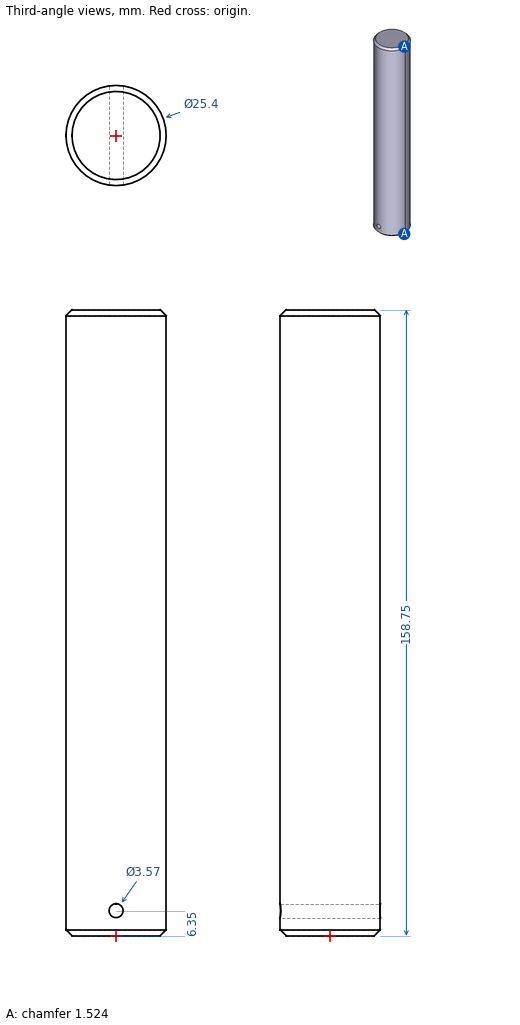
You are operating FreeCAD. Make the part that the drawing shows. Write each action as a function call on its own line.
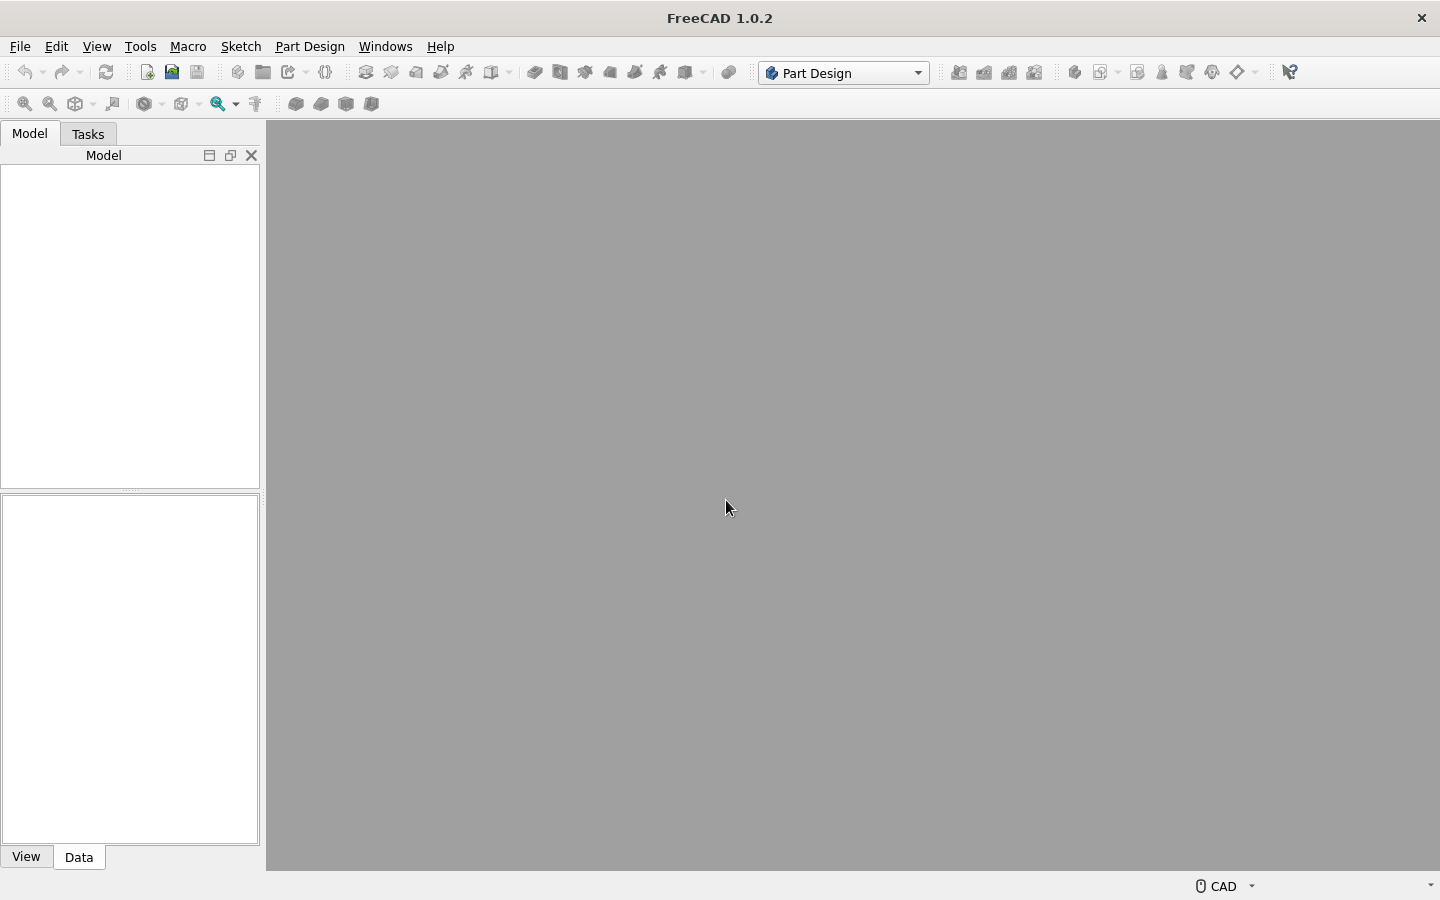
key(ctrl+n)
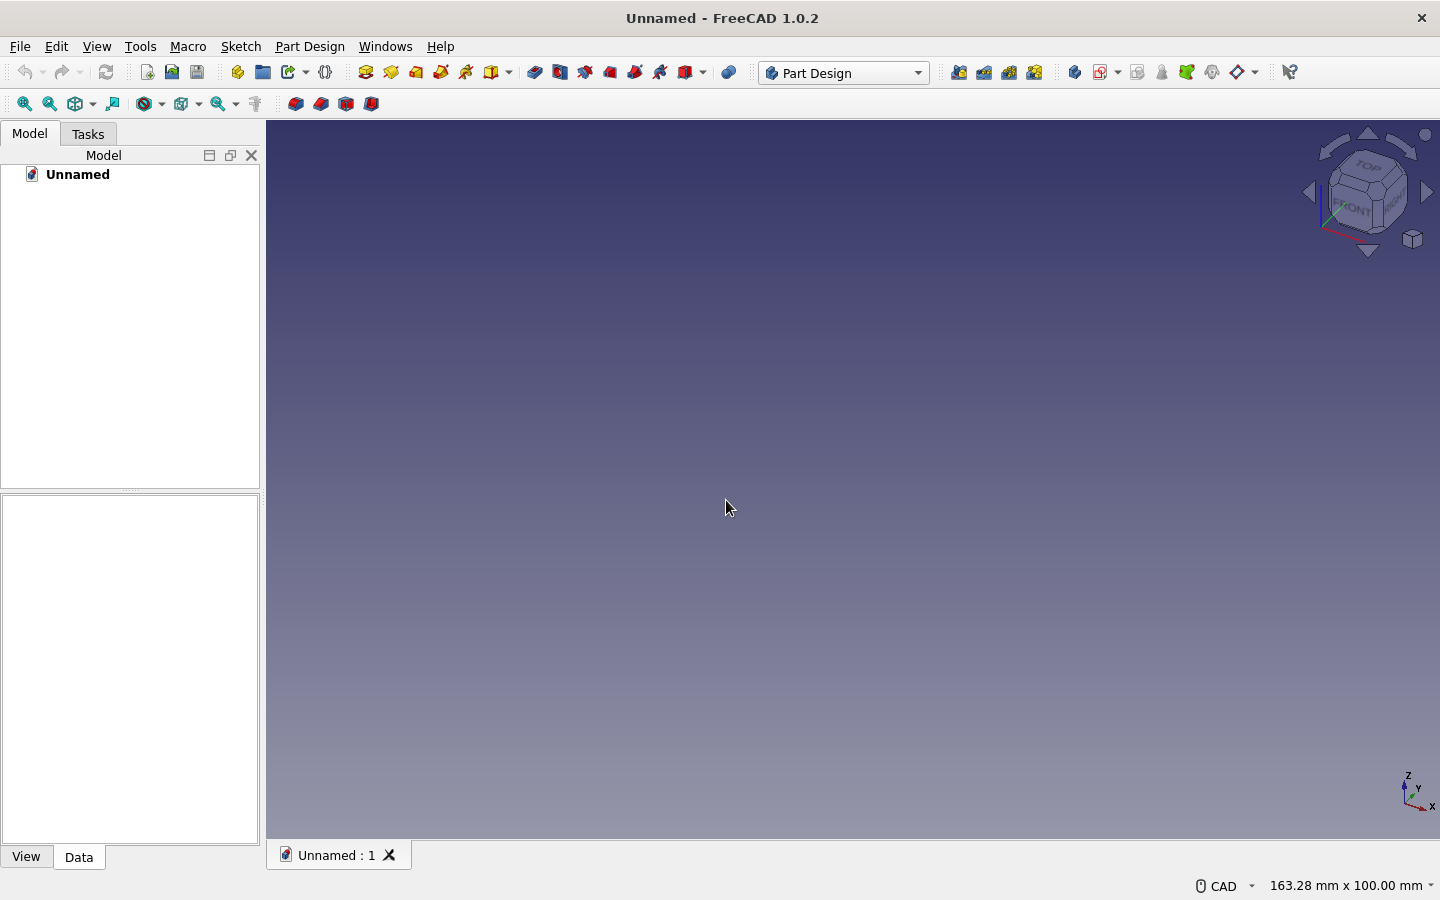
click(1100, 72)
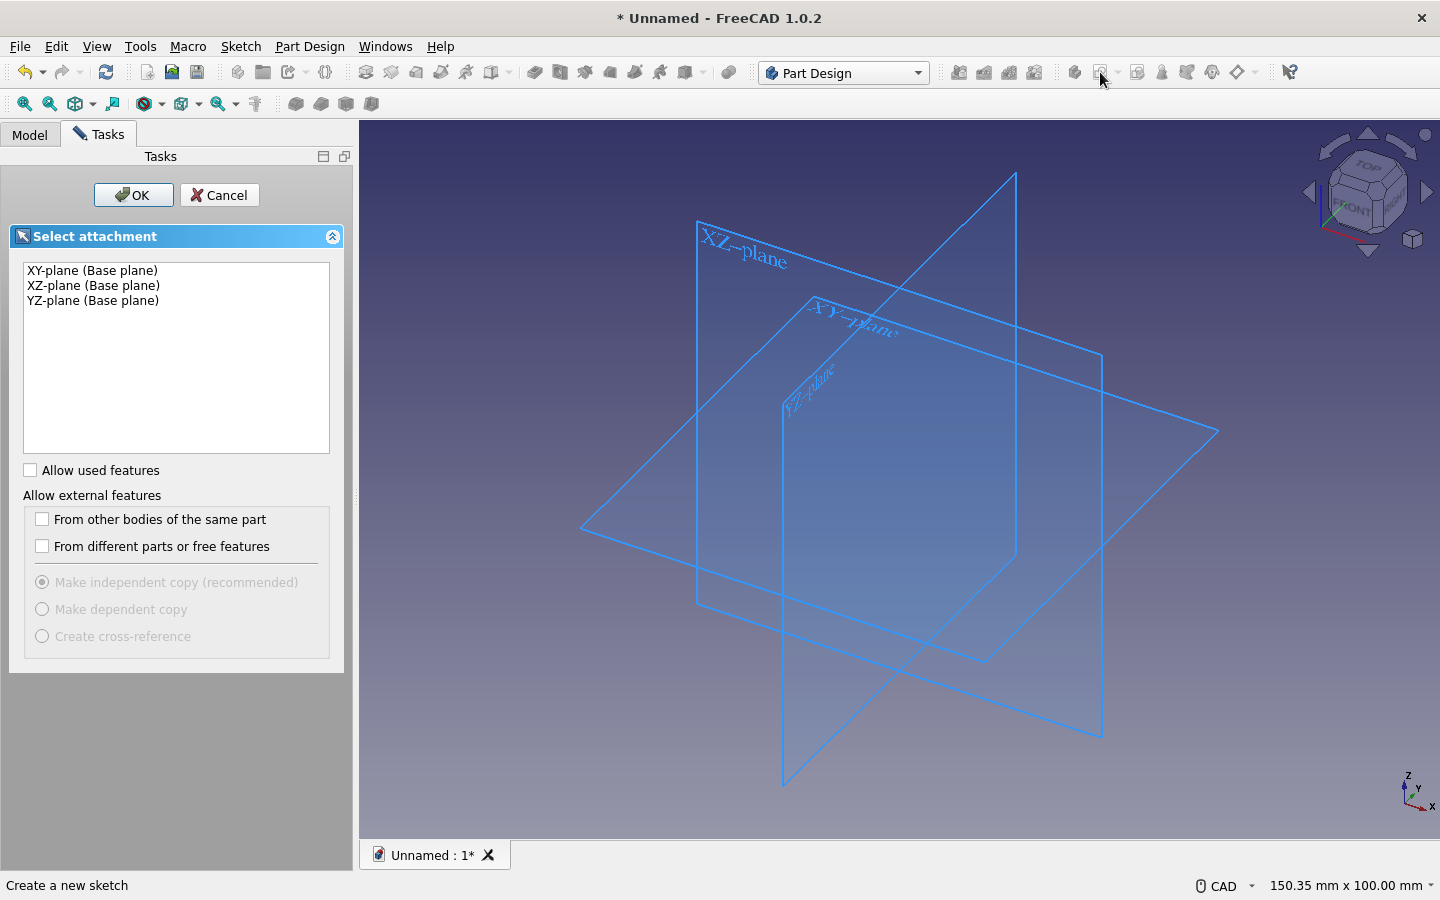
click(84, 270)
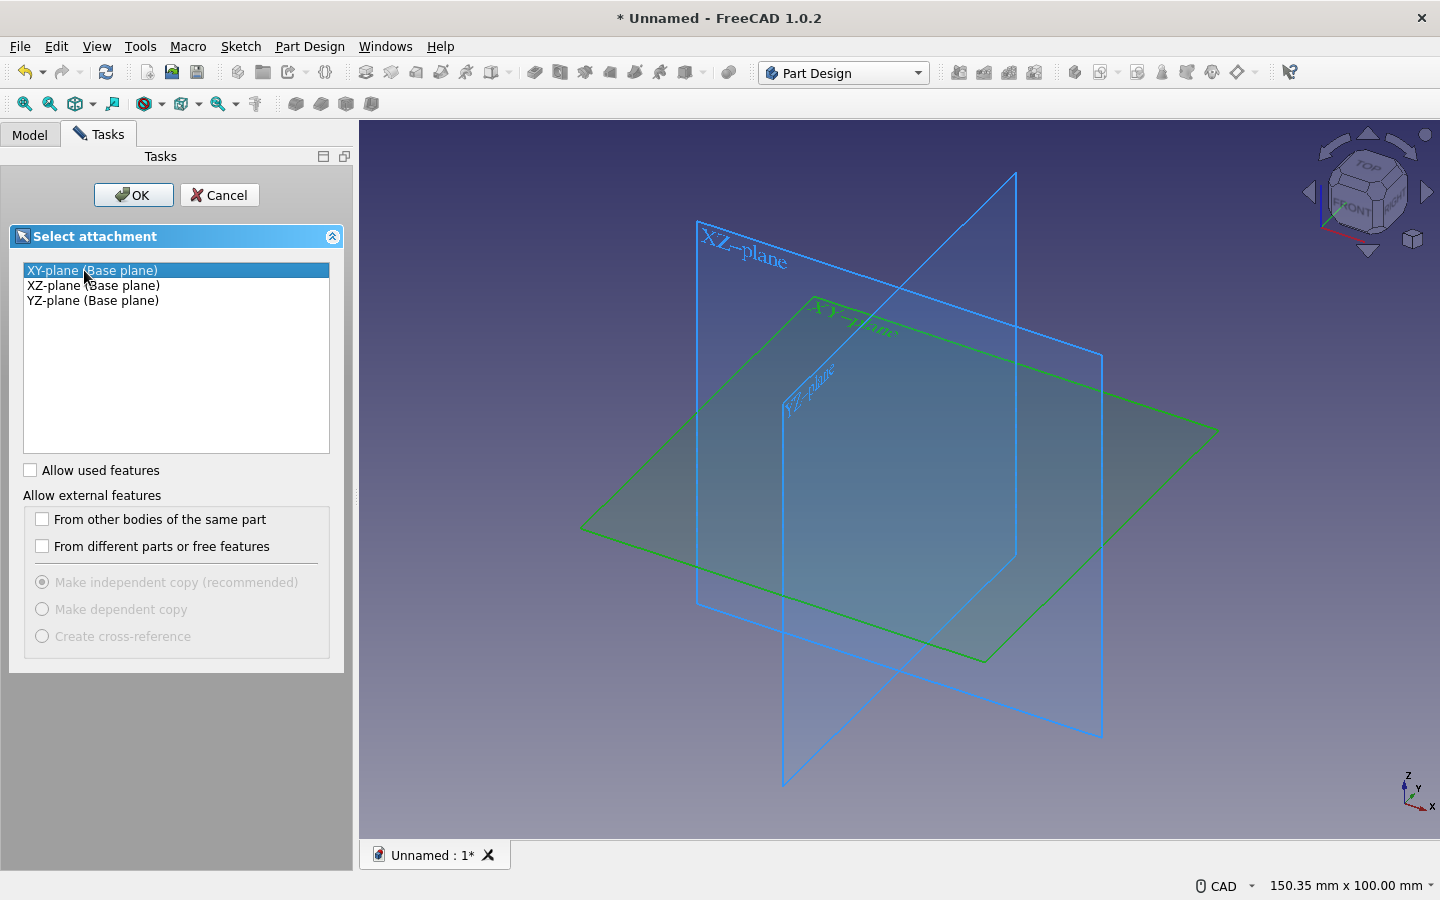
click(134, 195)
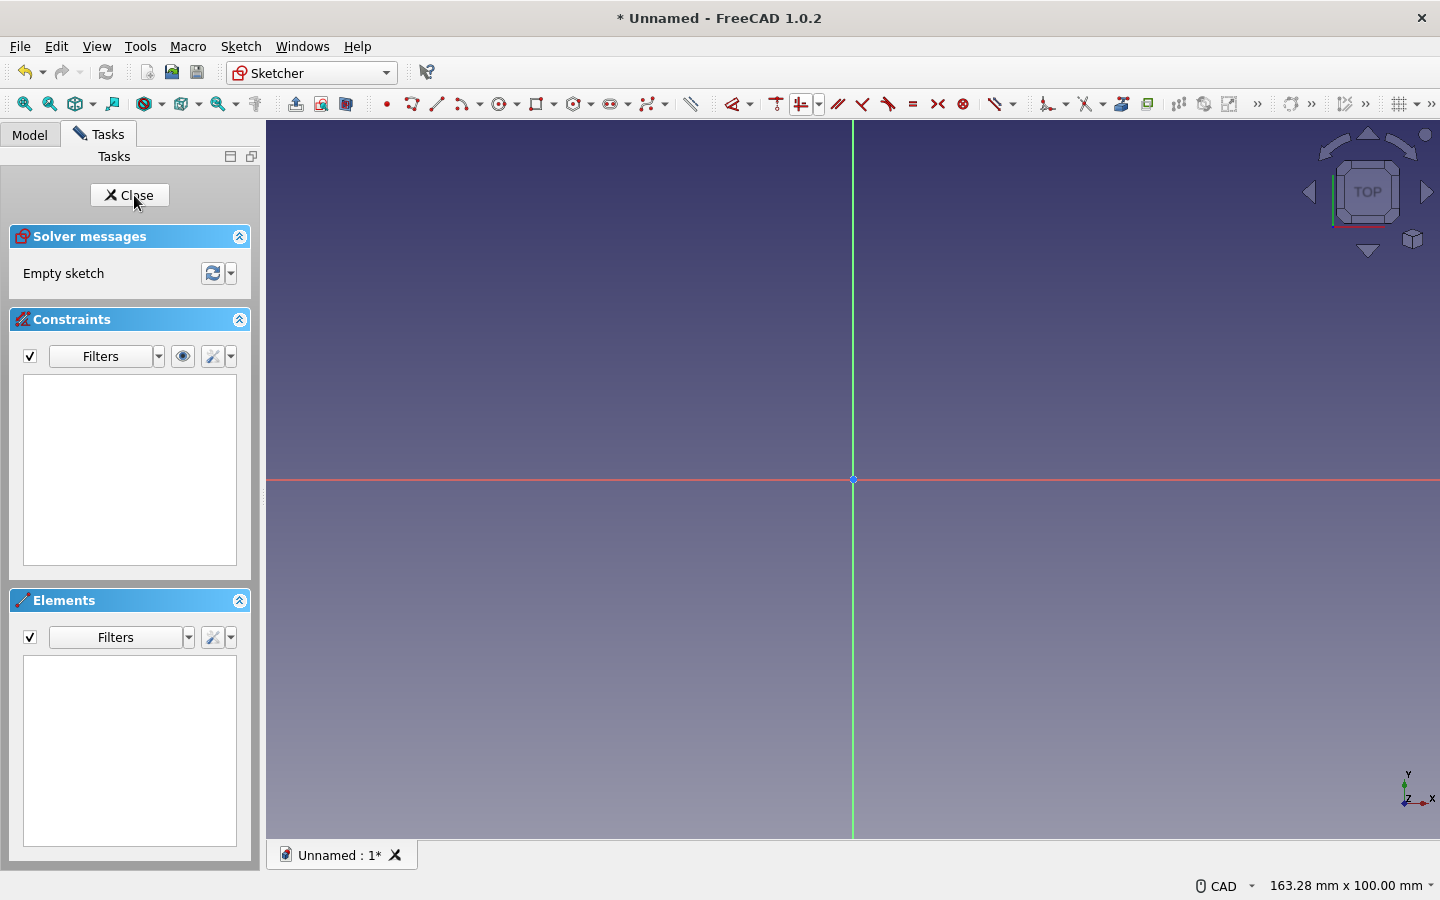
scroll(893, 480, up, 5)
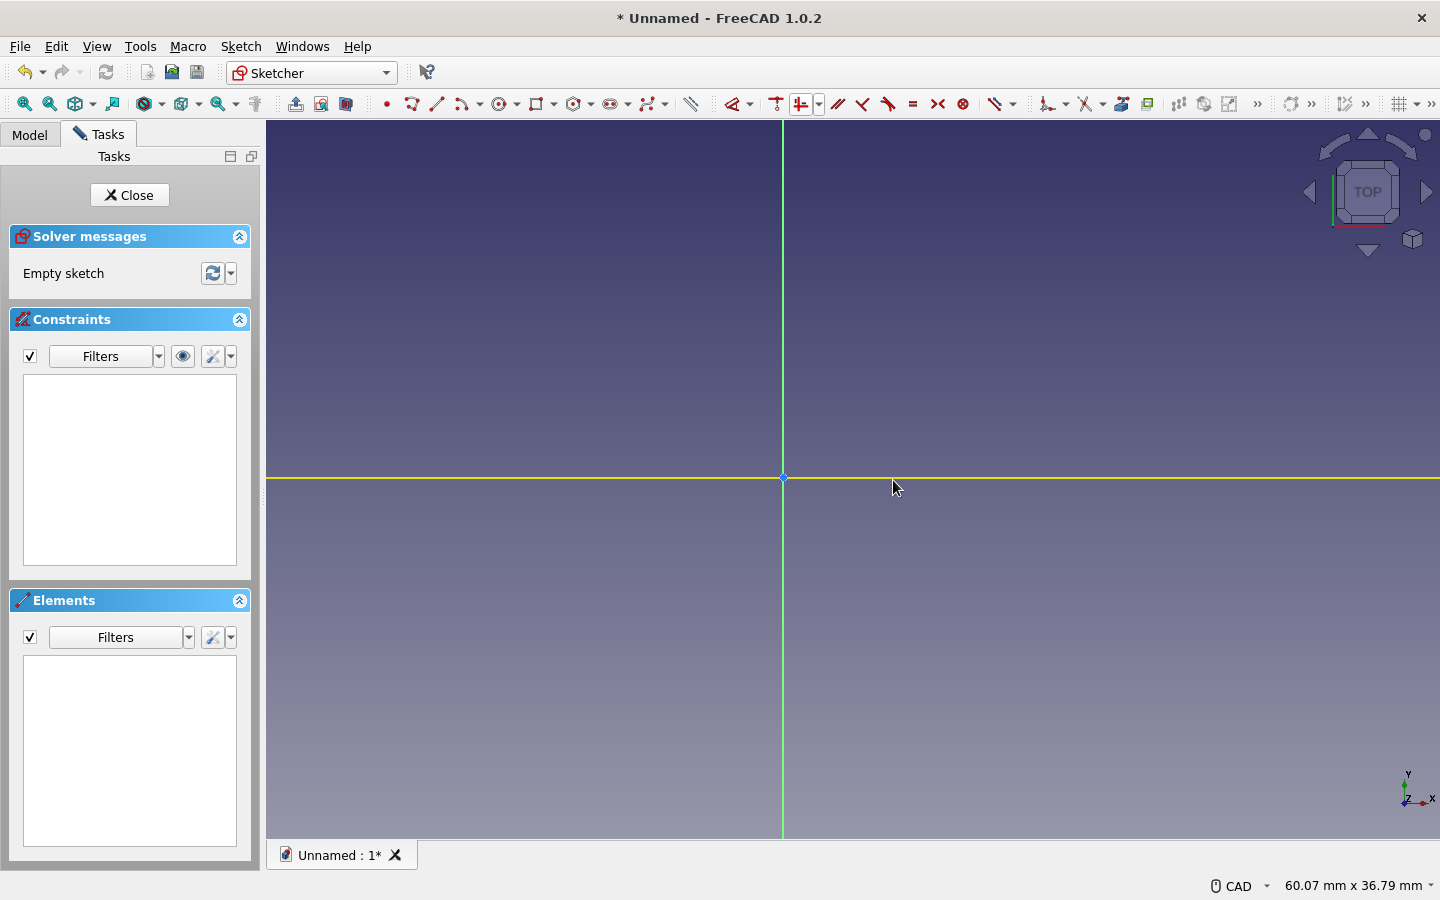
key(g)
key(c)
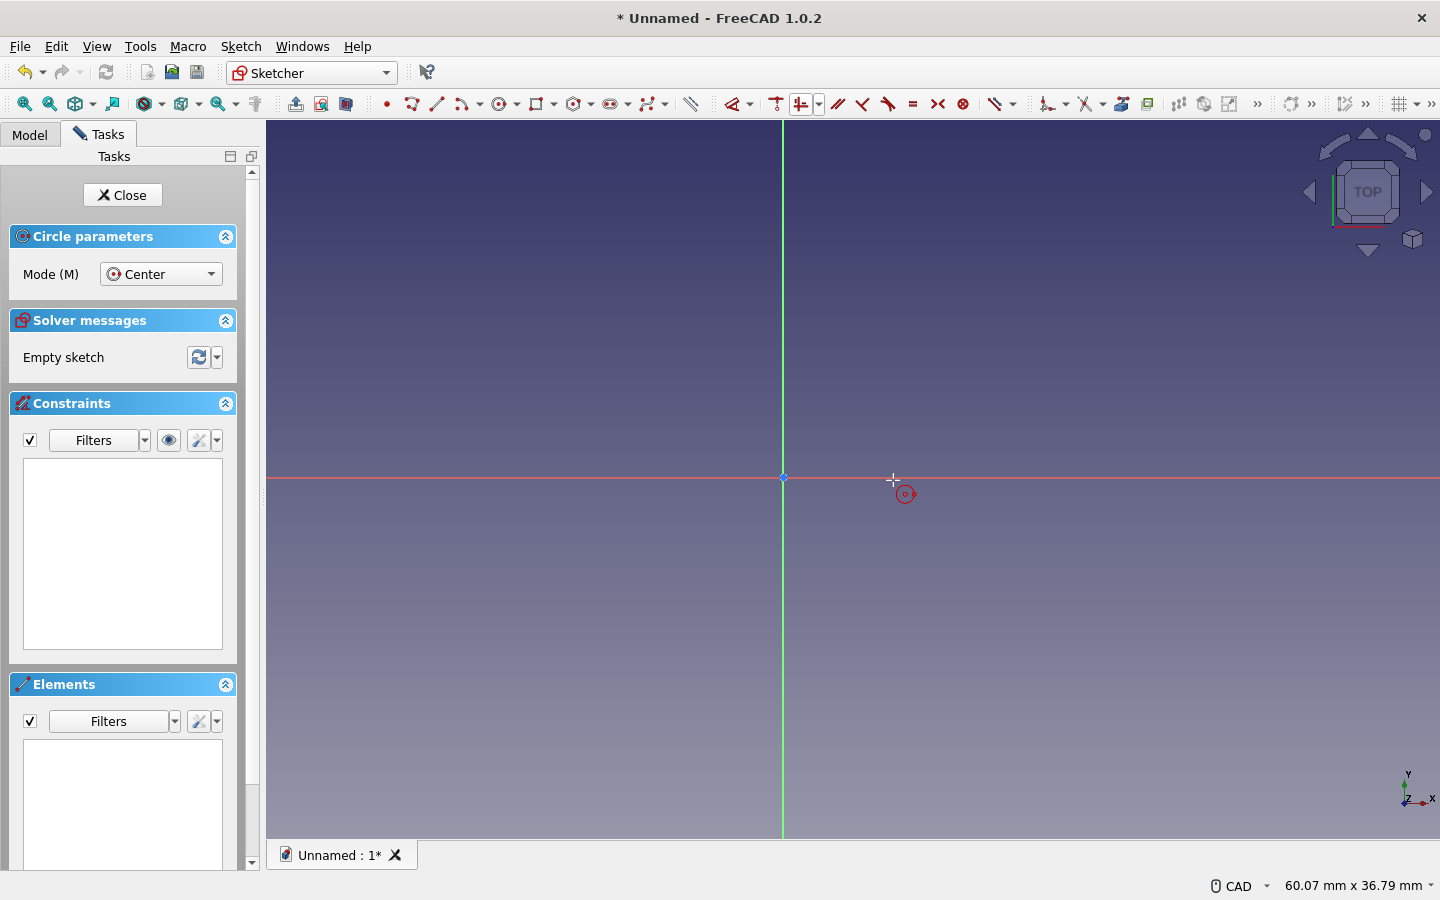
click(783, 478)
click(959, 302)
key(Escape)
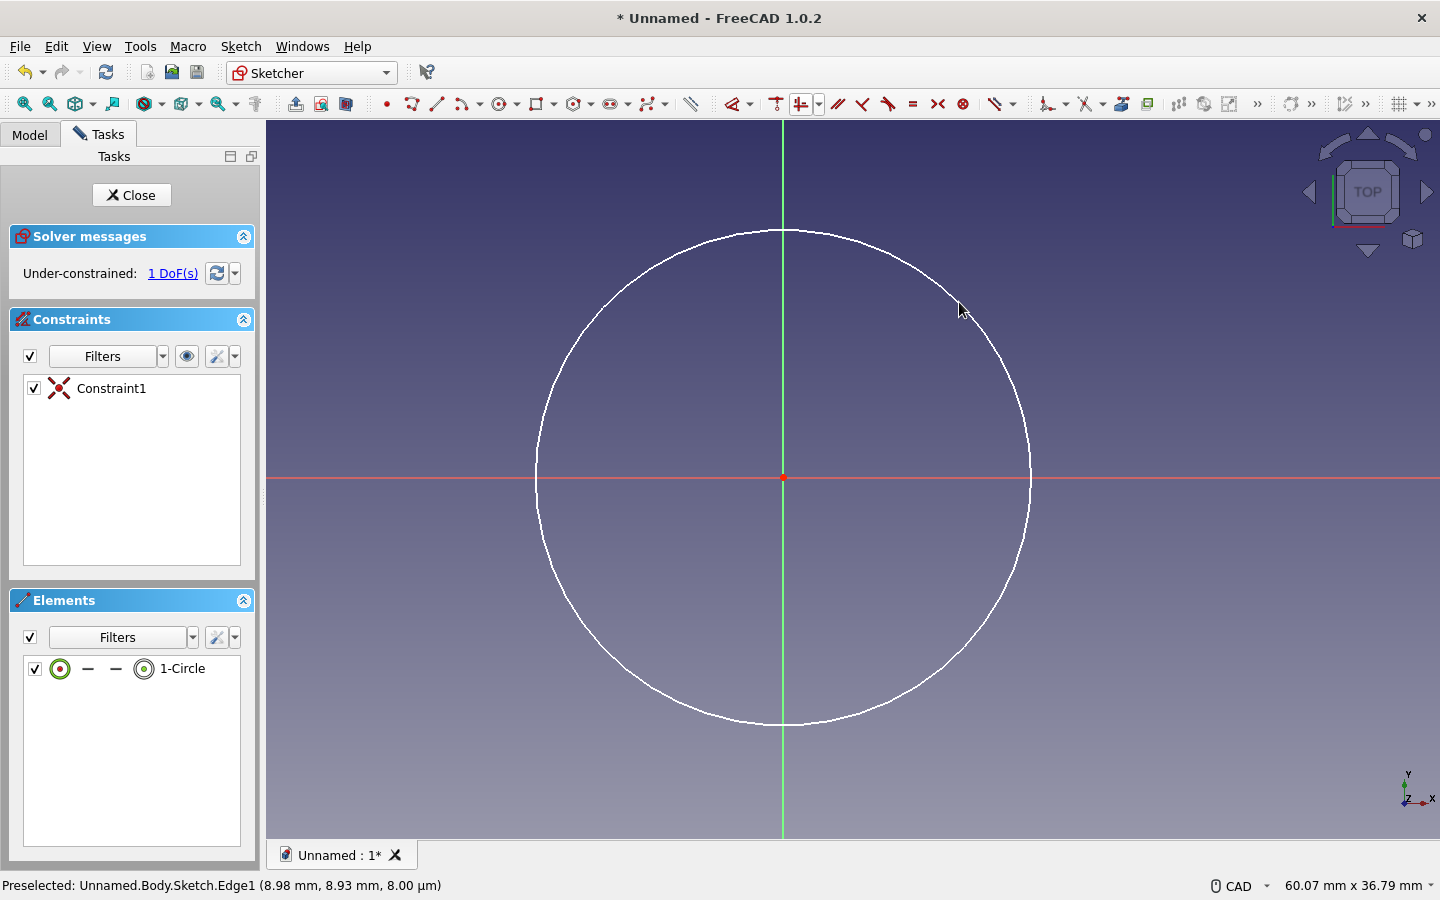
click(958, 302)